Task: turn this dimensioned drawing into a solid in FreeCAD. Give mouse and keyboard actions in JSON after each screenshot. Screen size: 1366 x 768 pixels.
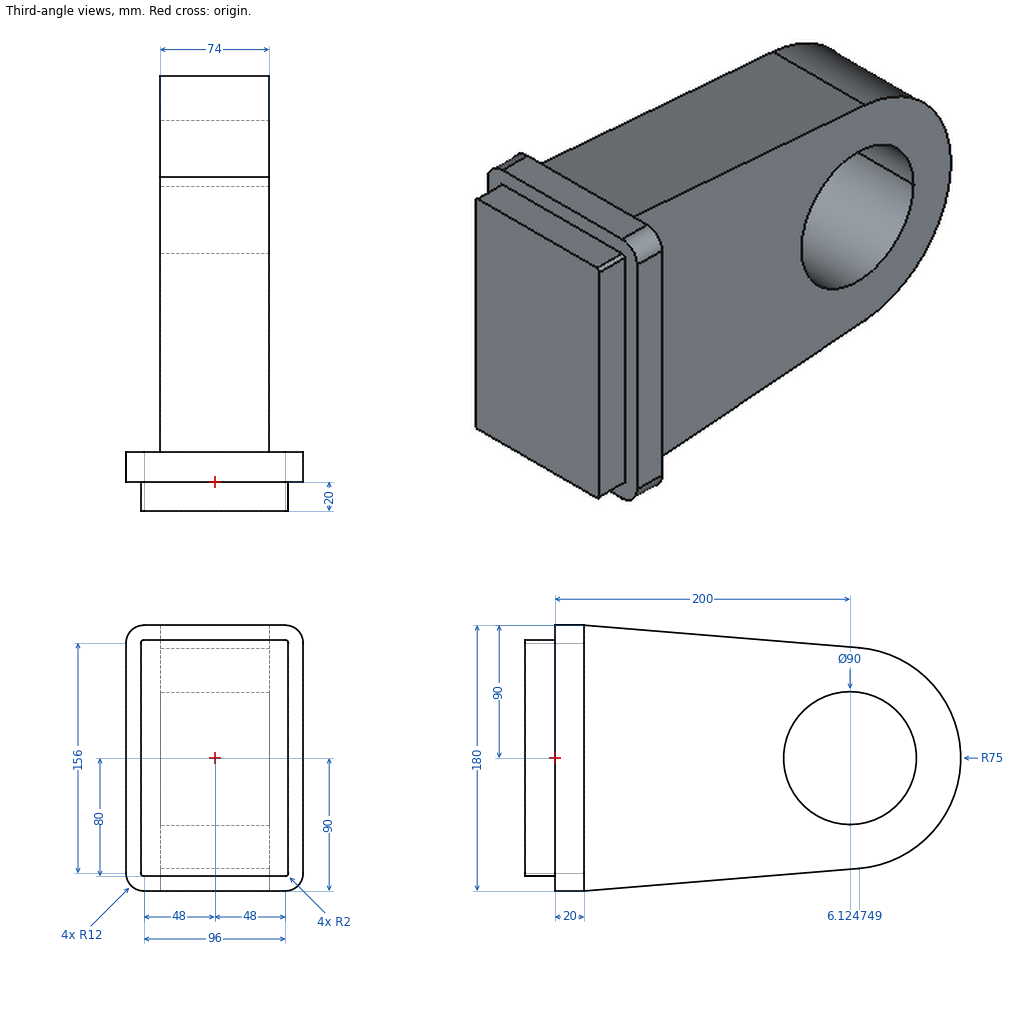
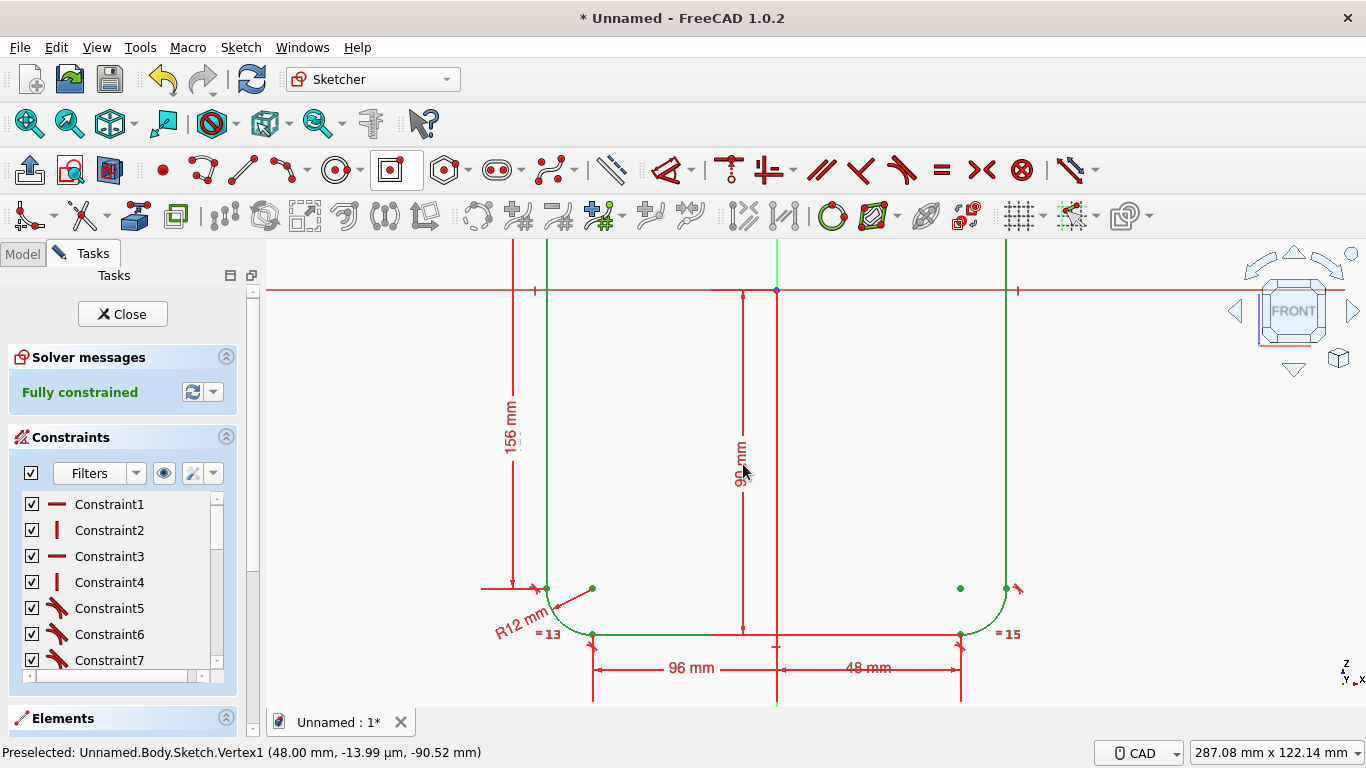
{"action": "left_click", "coordinate": [123, 314]}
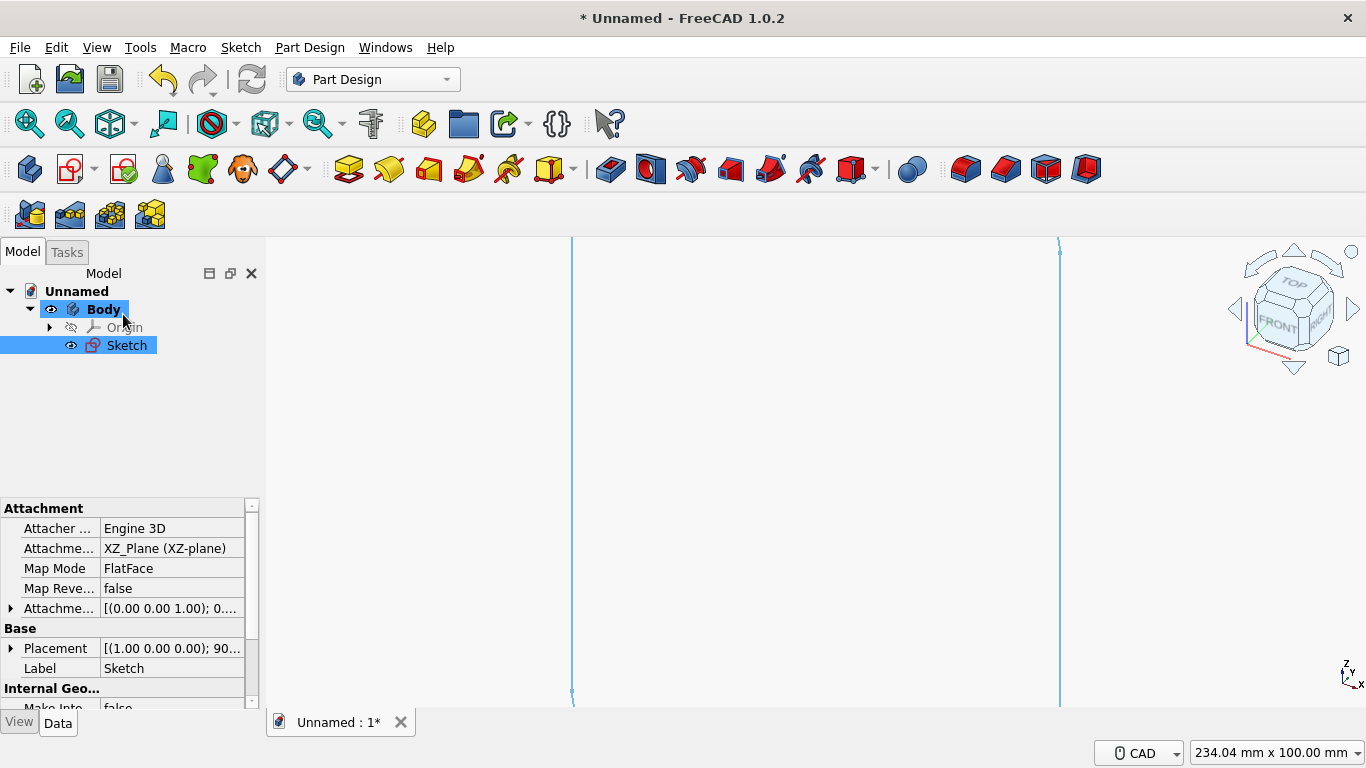
{"action": "left_click", "coordinate": [350, 170]}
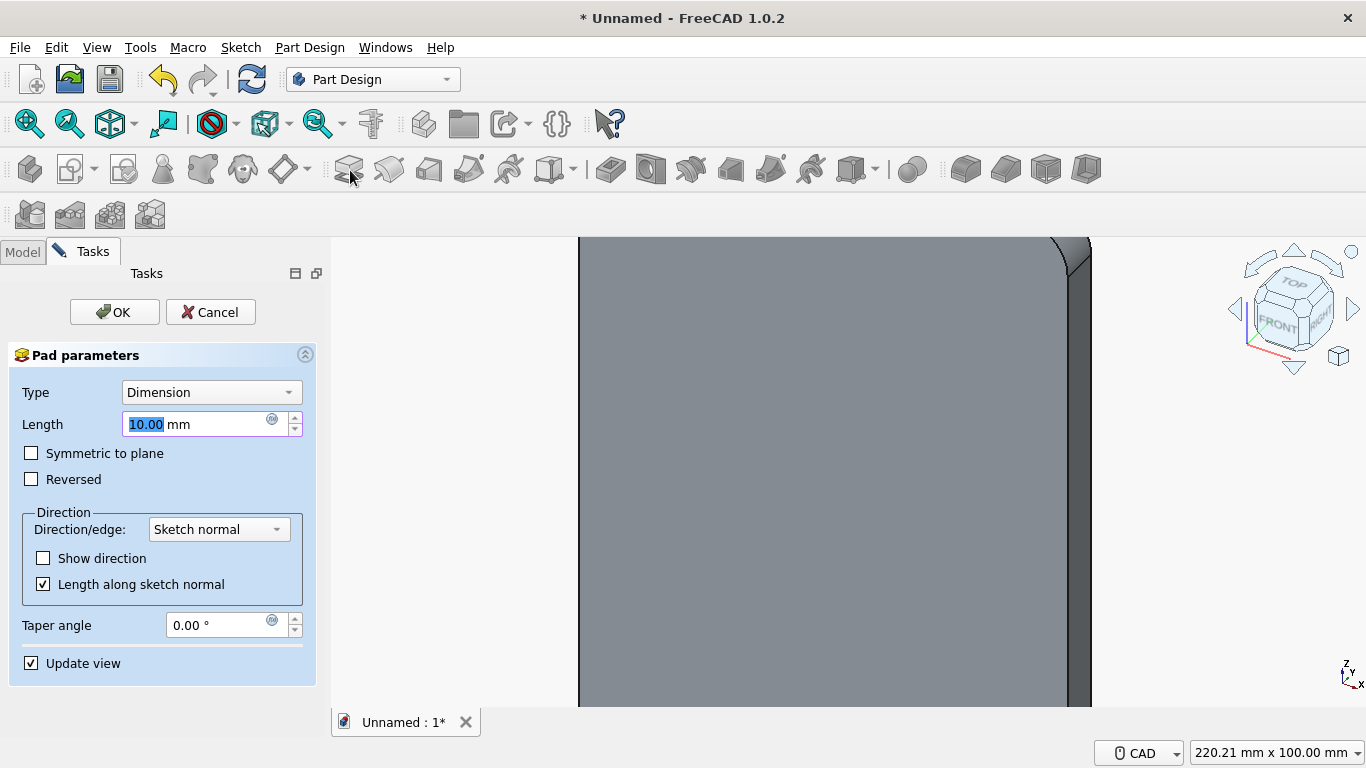
{"action": "type", "text": "20"}
{"action": "key", "text": "Tab"}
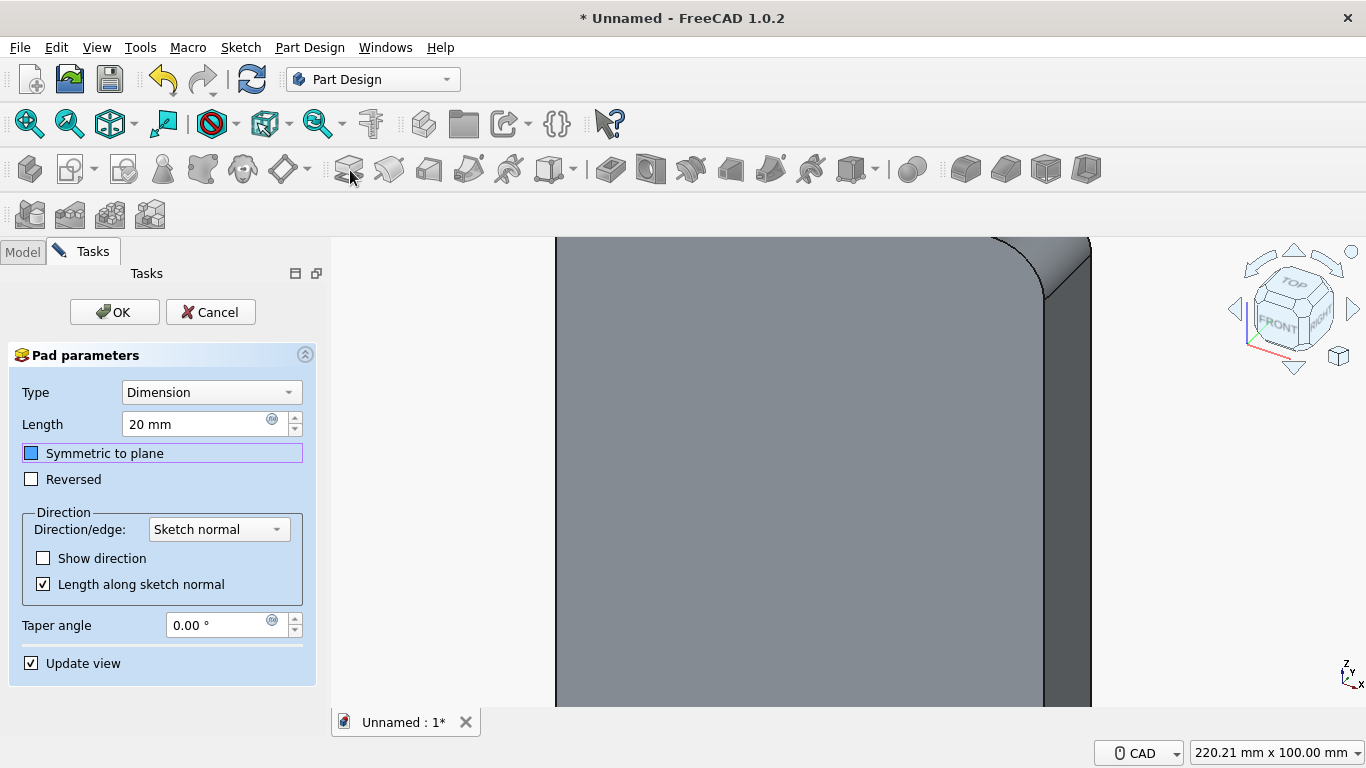
{"action": "left_click", "coordinate": [30, 479]}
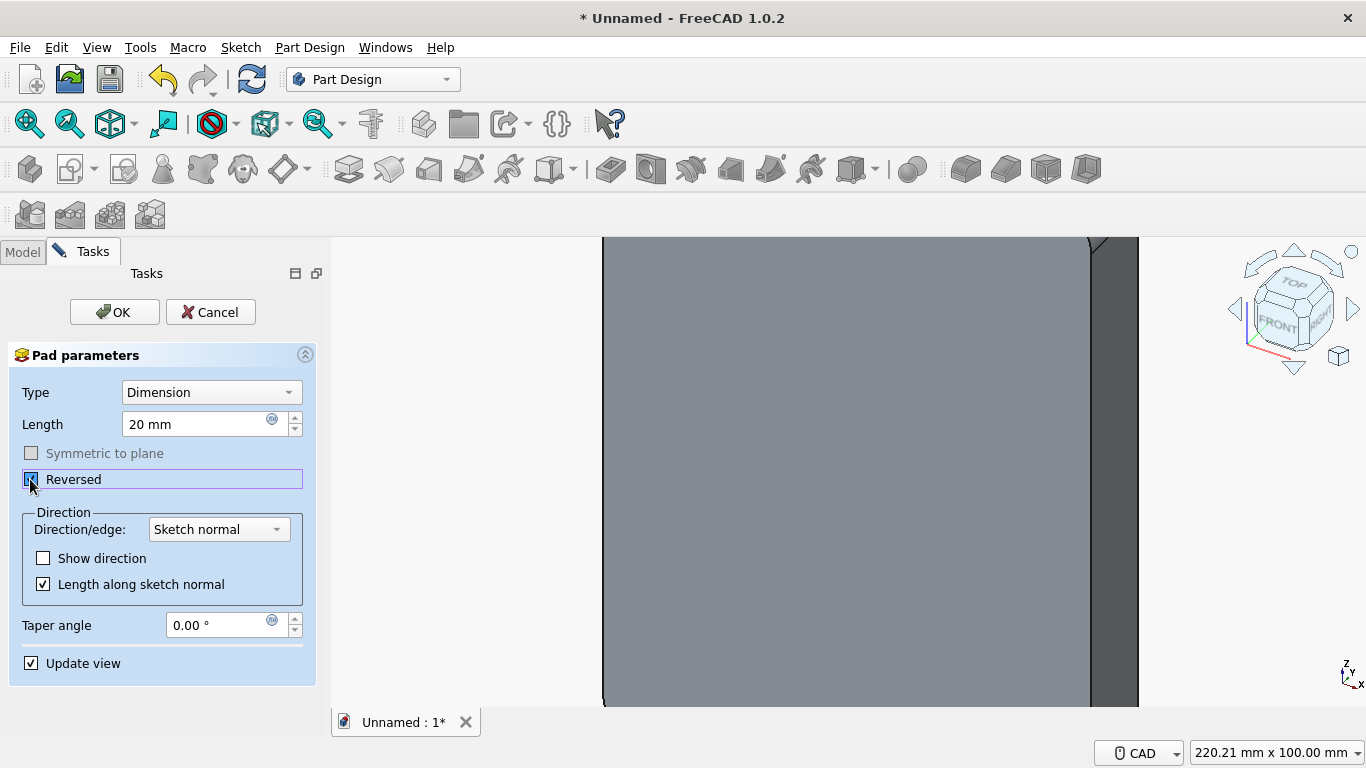
{"action": "left_click", "coordinate": [115, 312]}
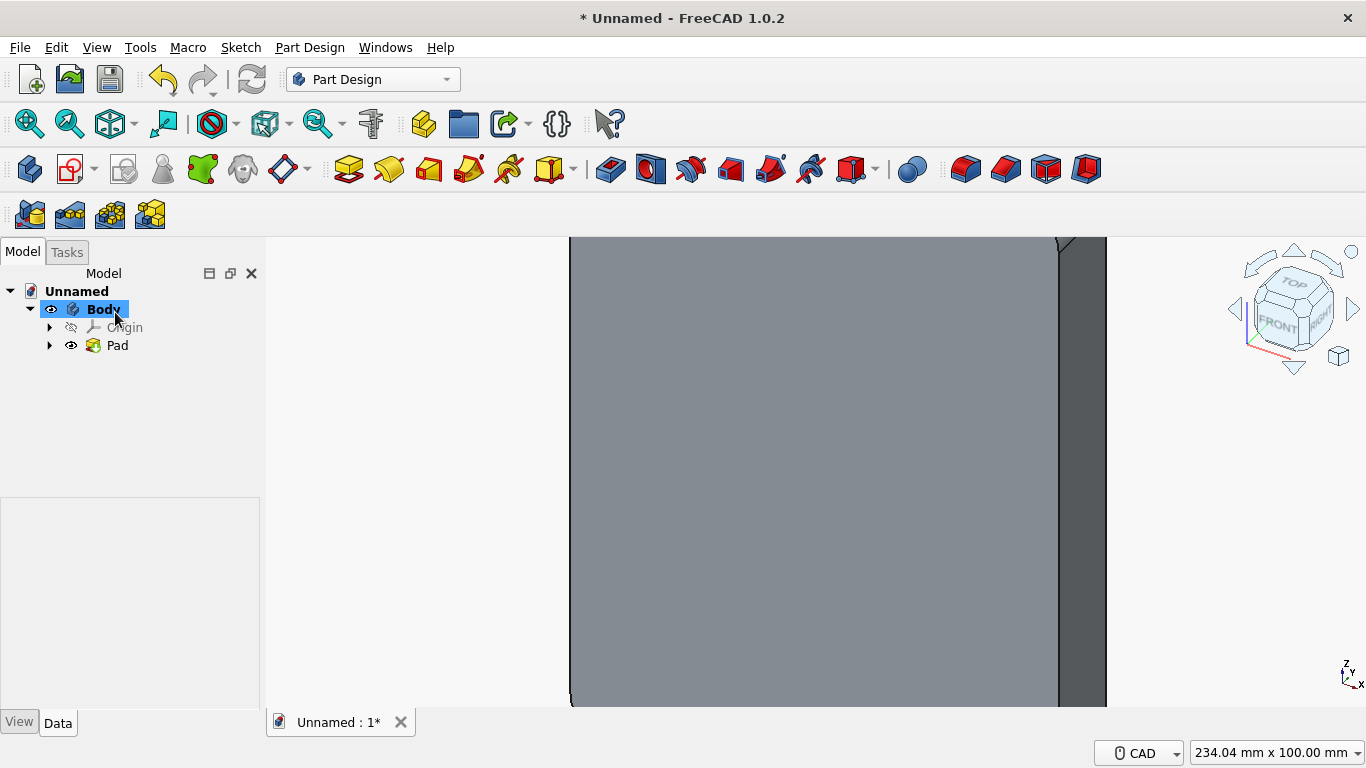
{"action": "key", "text": "v f"}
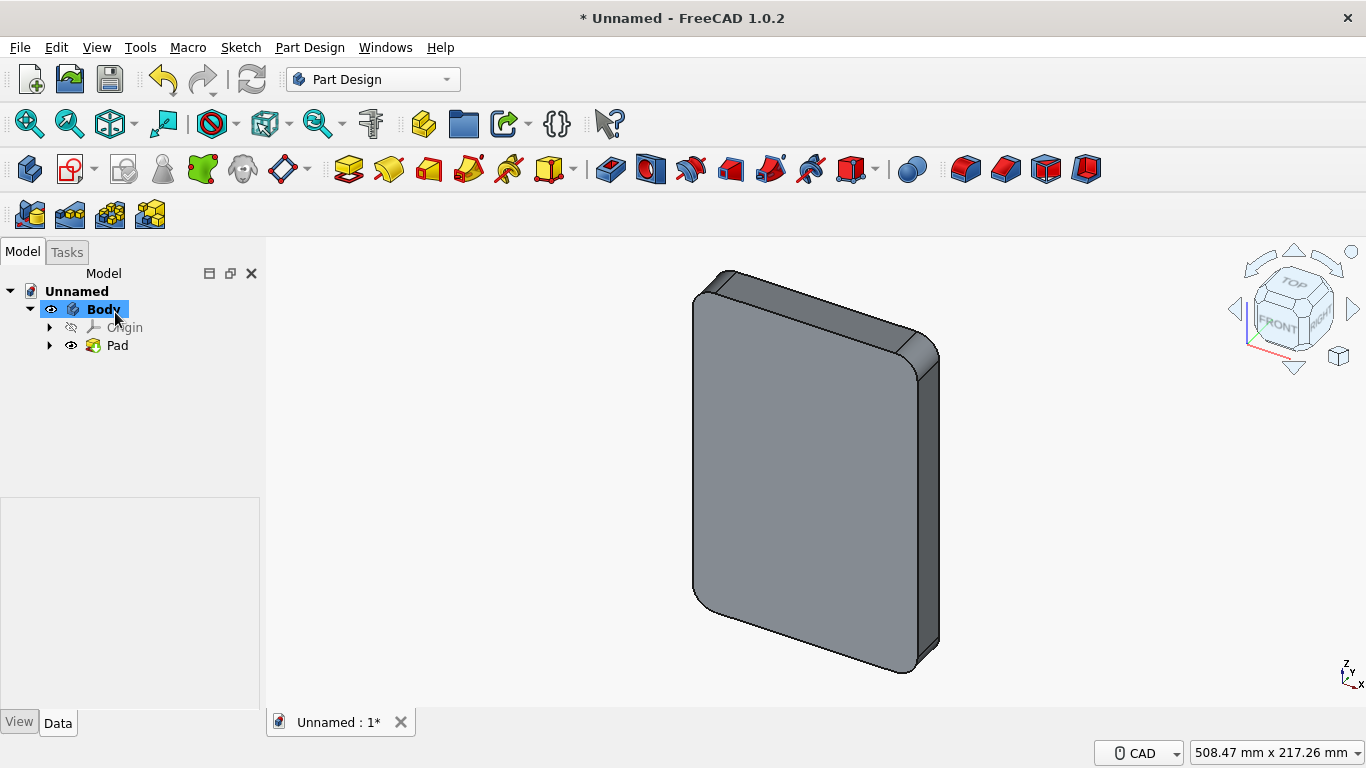
{"action": "left_click", "coordinate": [805, 436]}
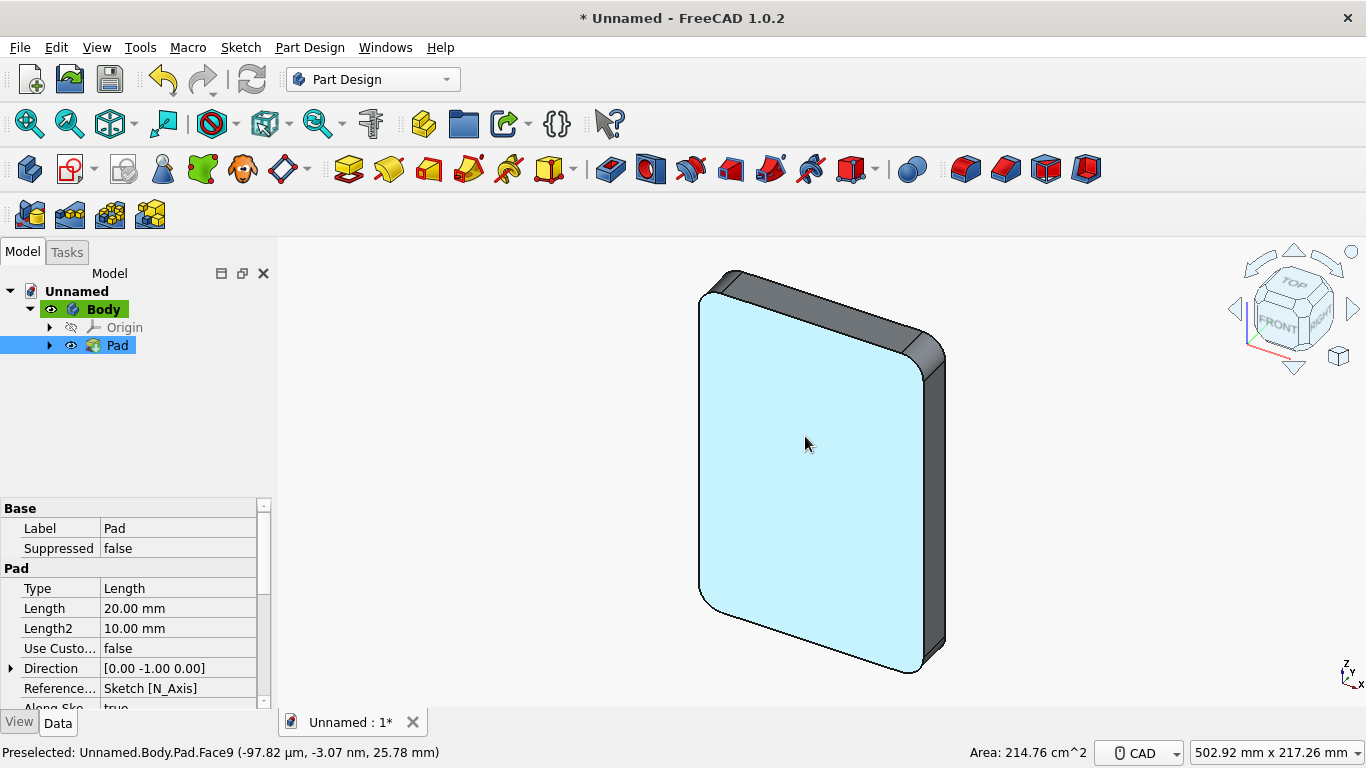
{"action": "left_click", "coordinate": [70, 170]}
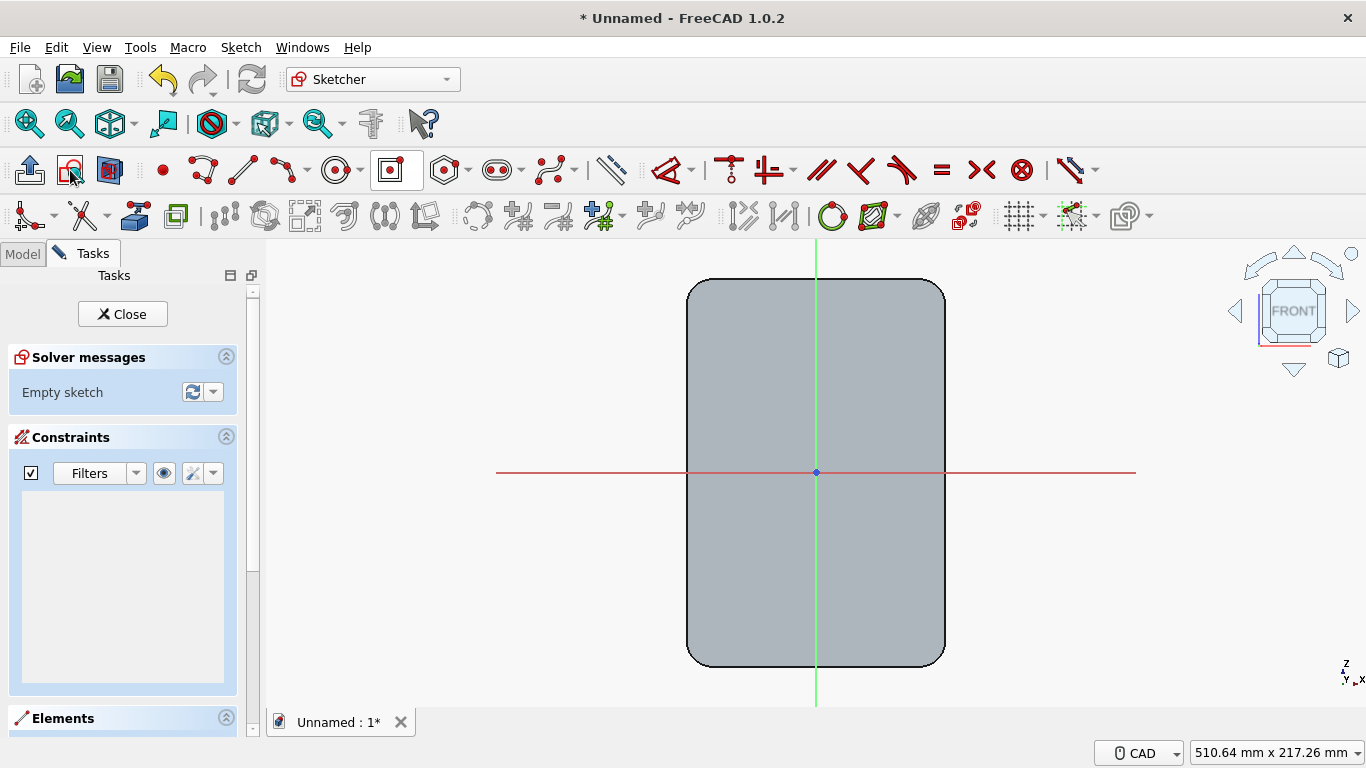
{"action": "key", "text": "g l"}